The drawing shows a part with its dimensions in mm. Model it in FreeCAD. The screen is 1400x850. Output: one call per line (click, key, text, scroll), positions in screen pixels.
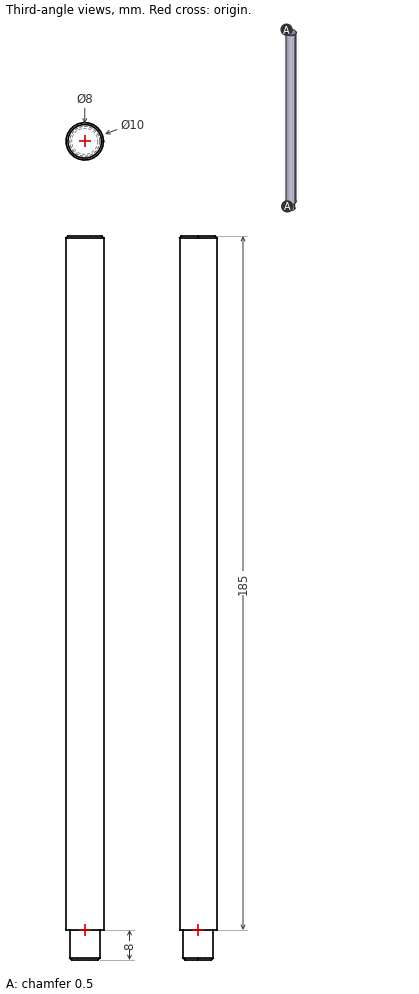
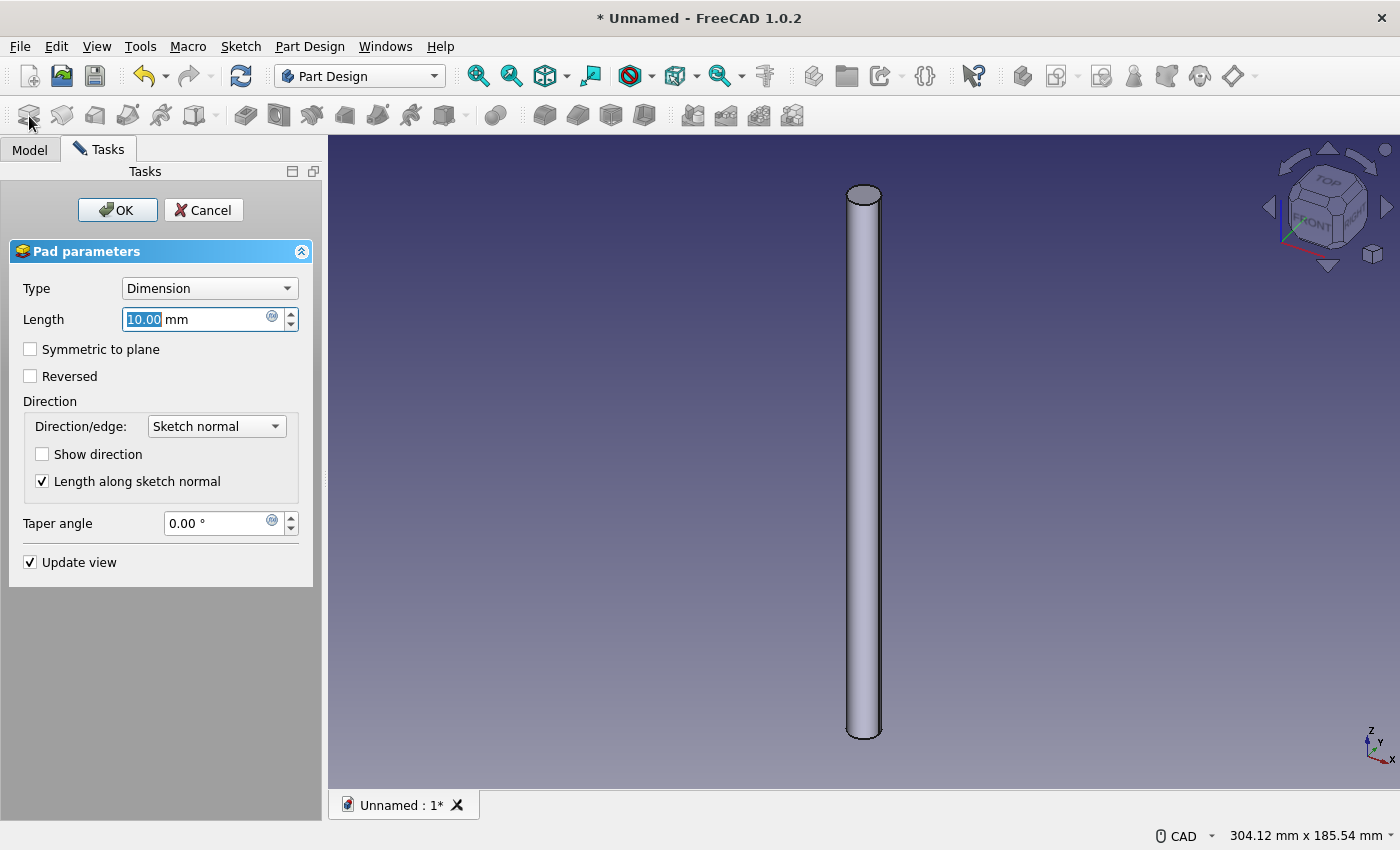
text(8)
key(Tab)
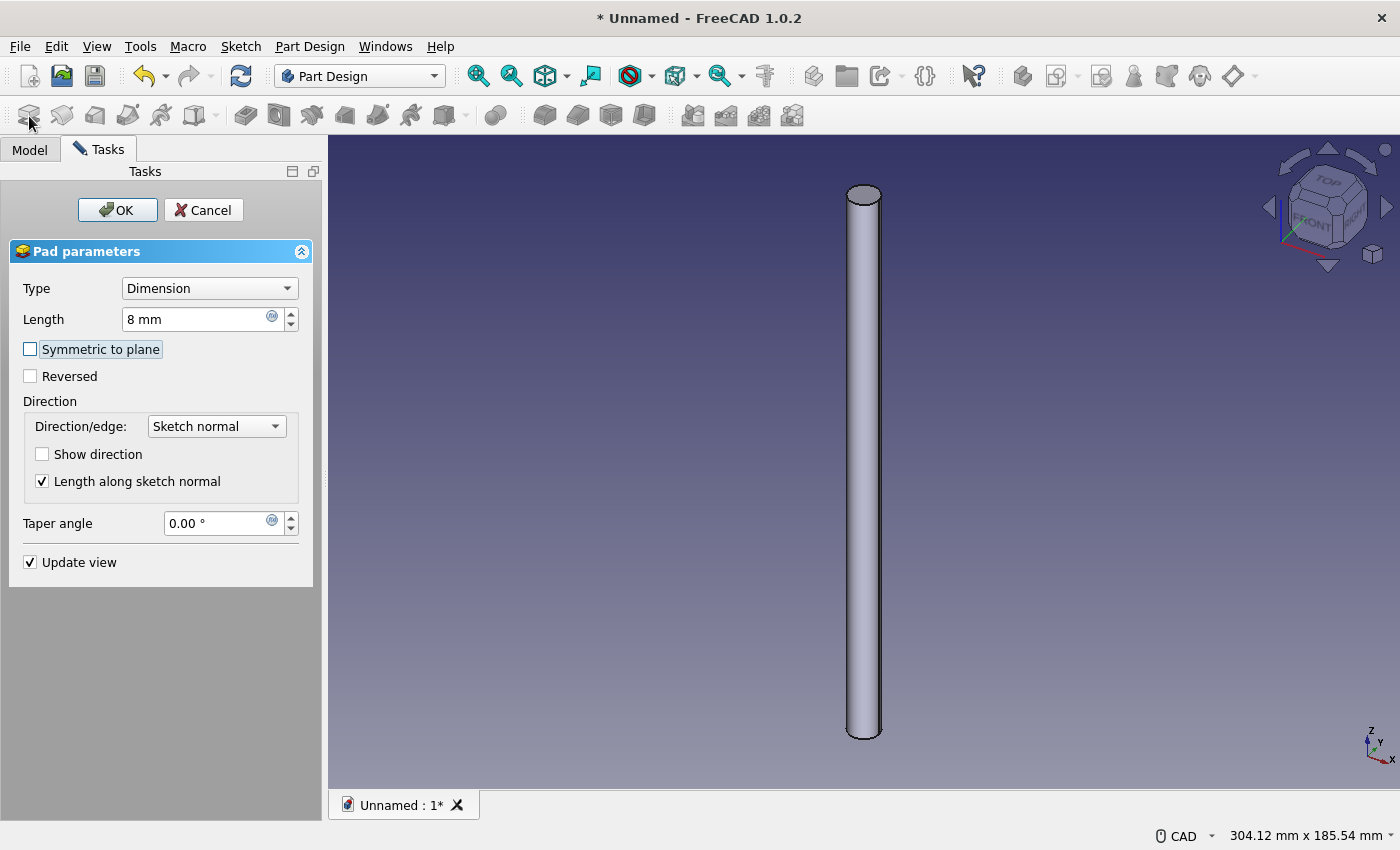
click(31, 376)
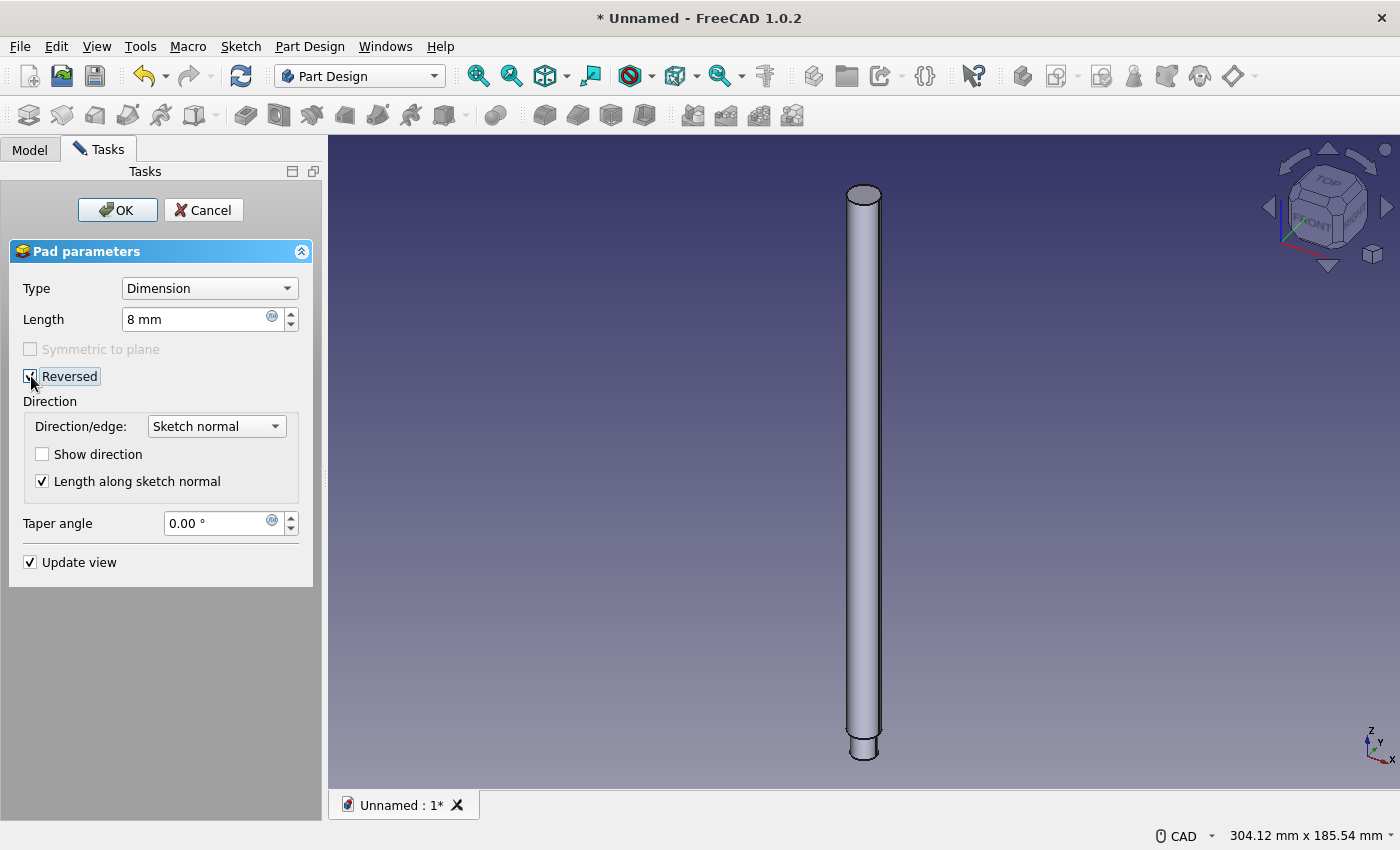
click(118, 210)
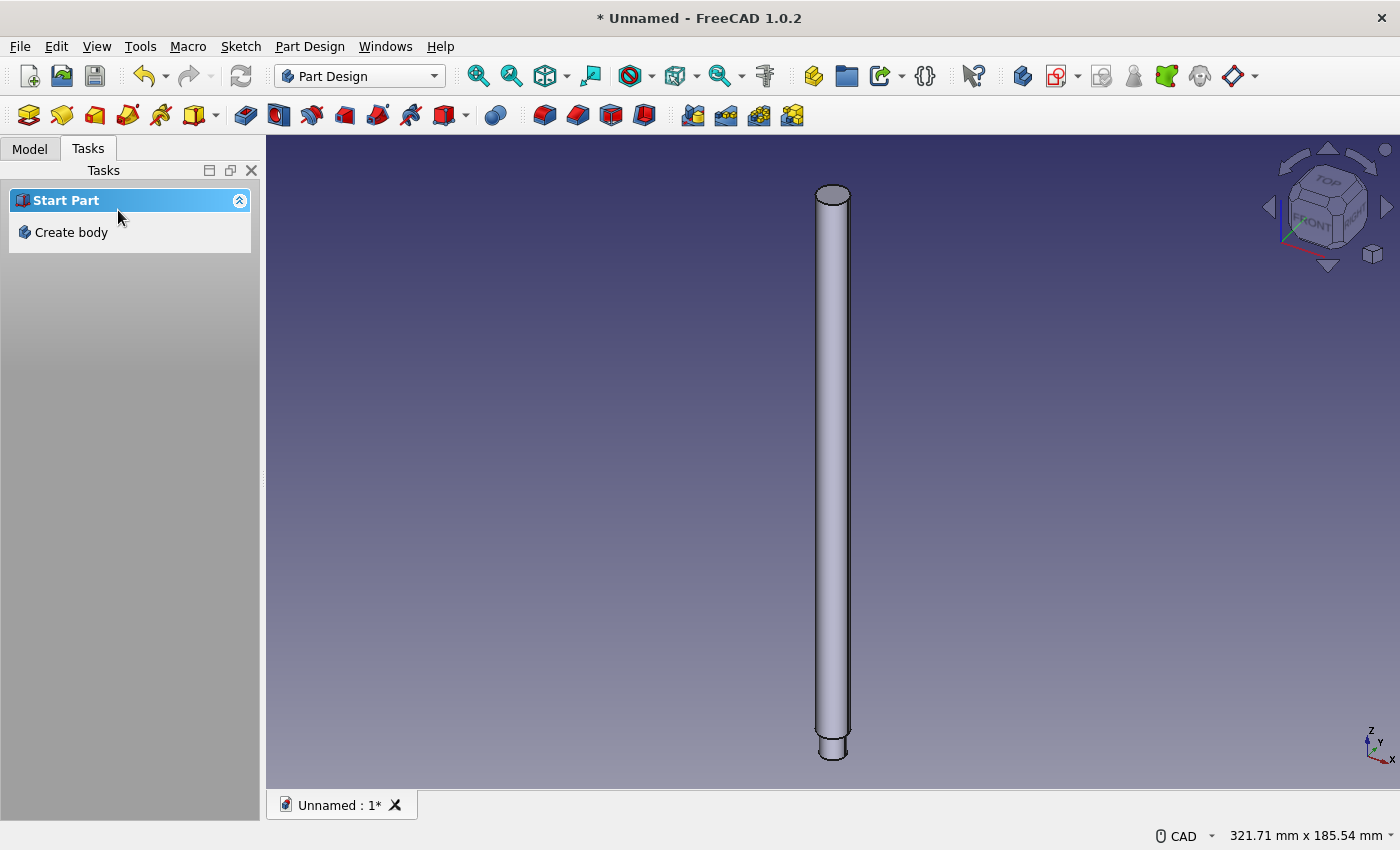
click(818, 189)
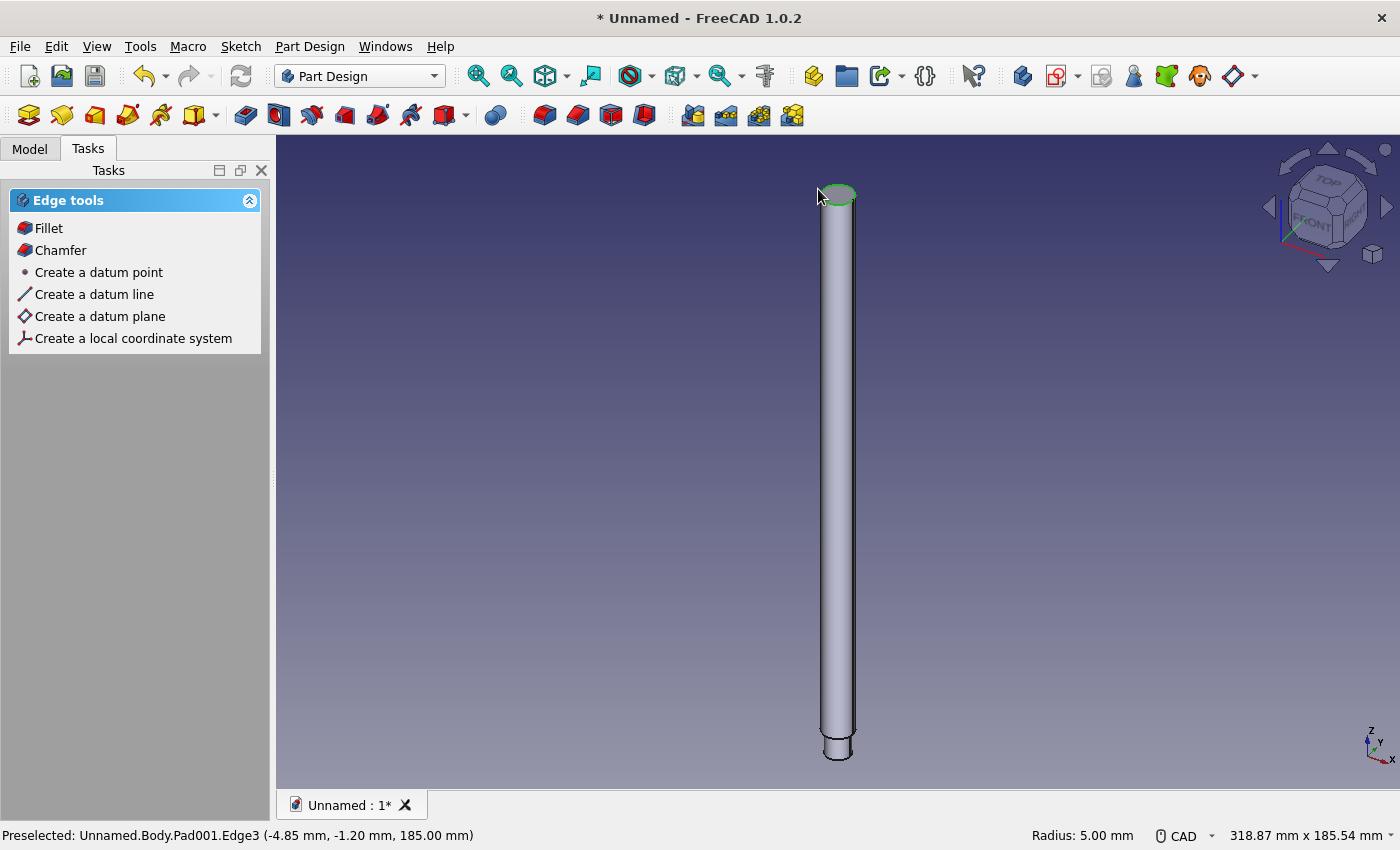
click(828, 757, ctrl)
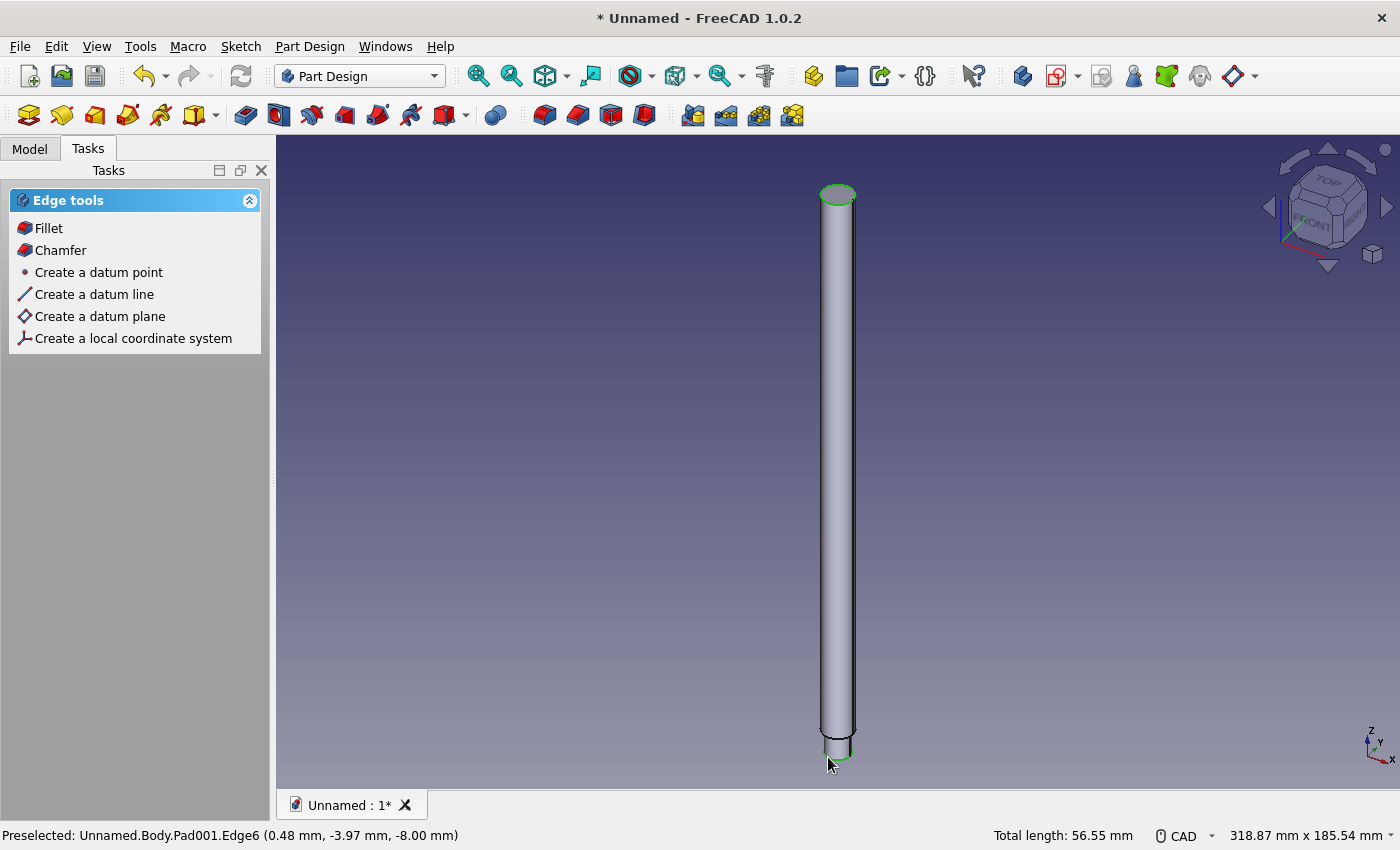
click(578, 116)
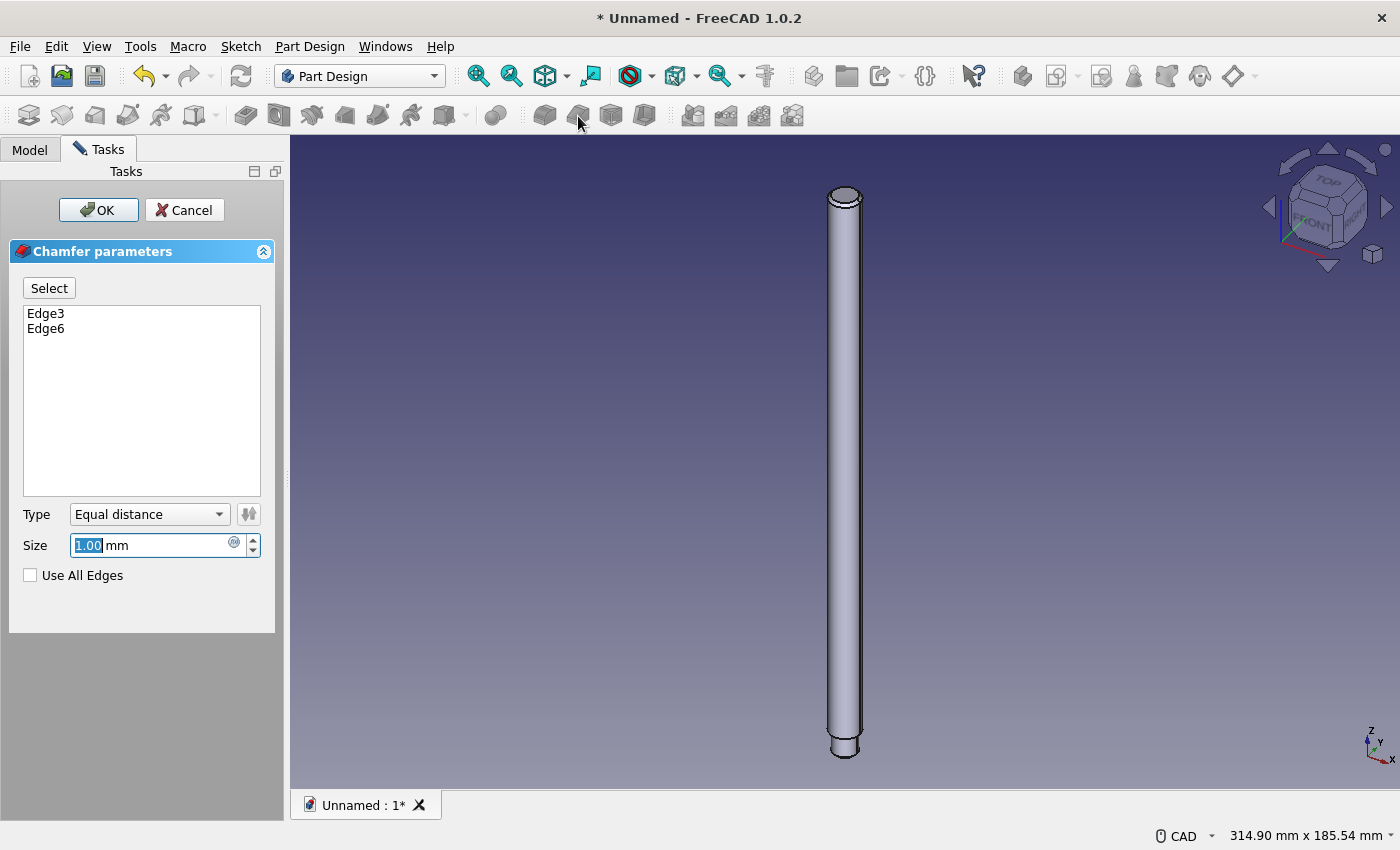
text(0.5)
key(Tab)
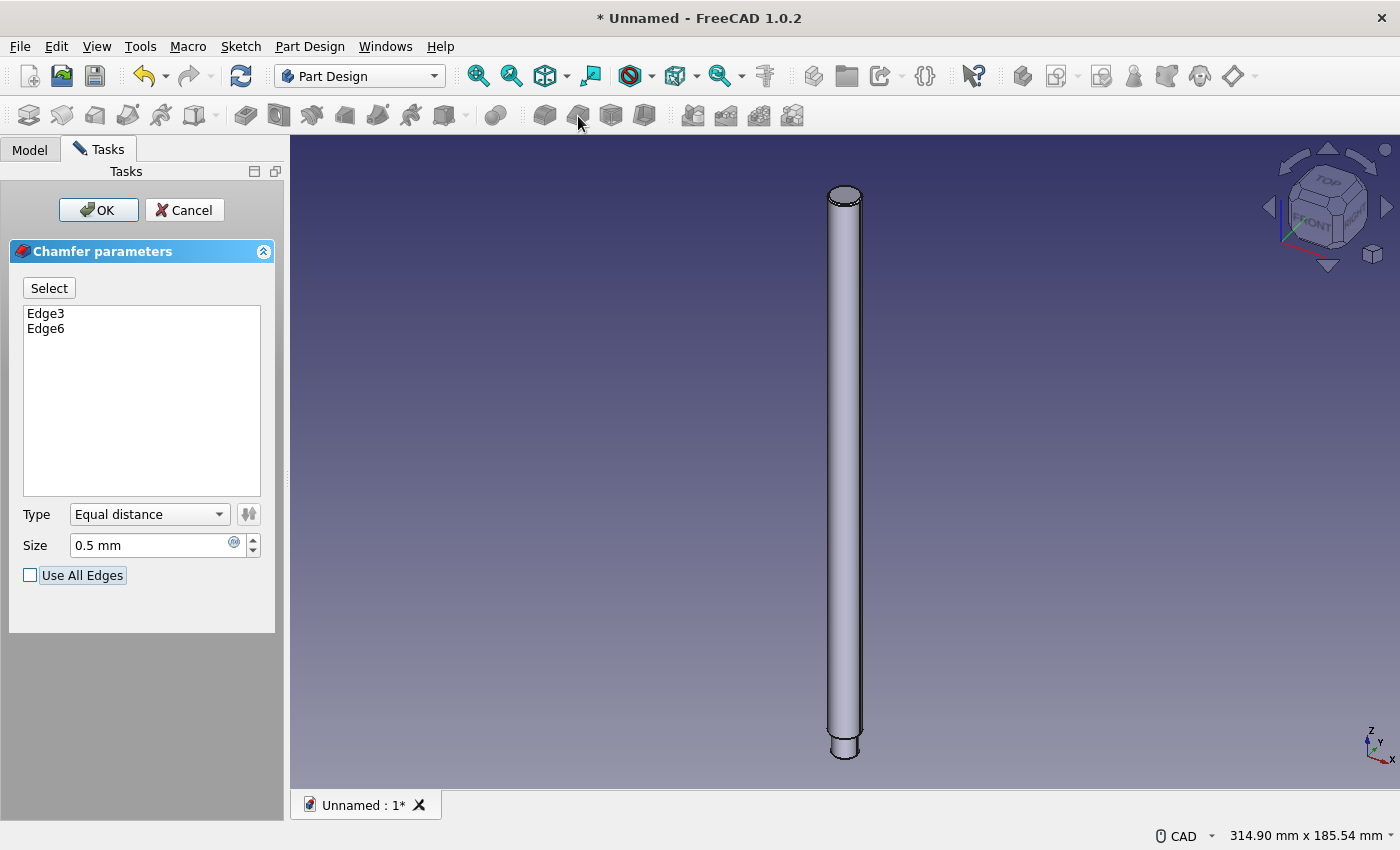
click(99, 210)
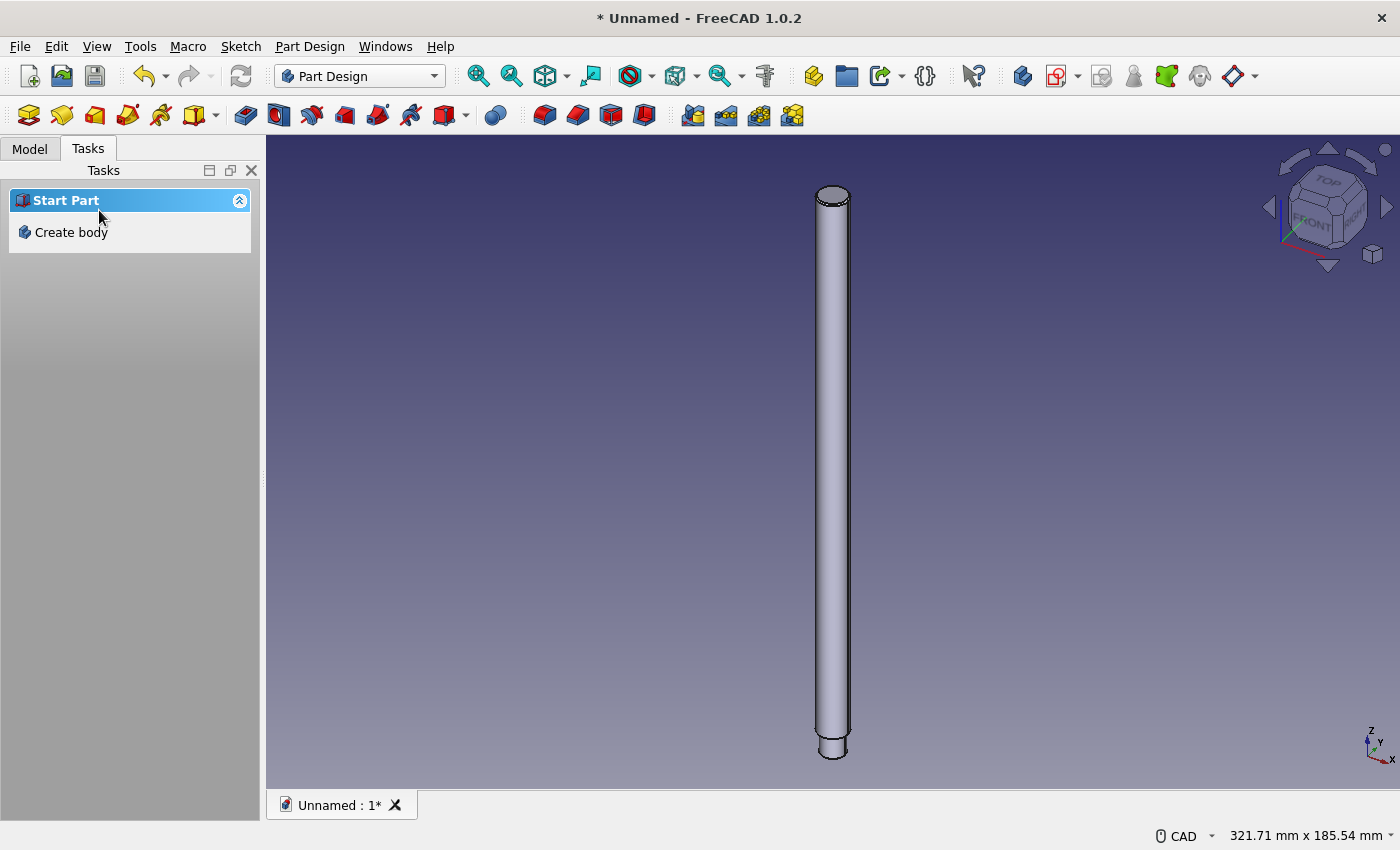
key(0)